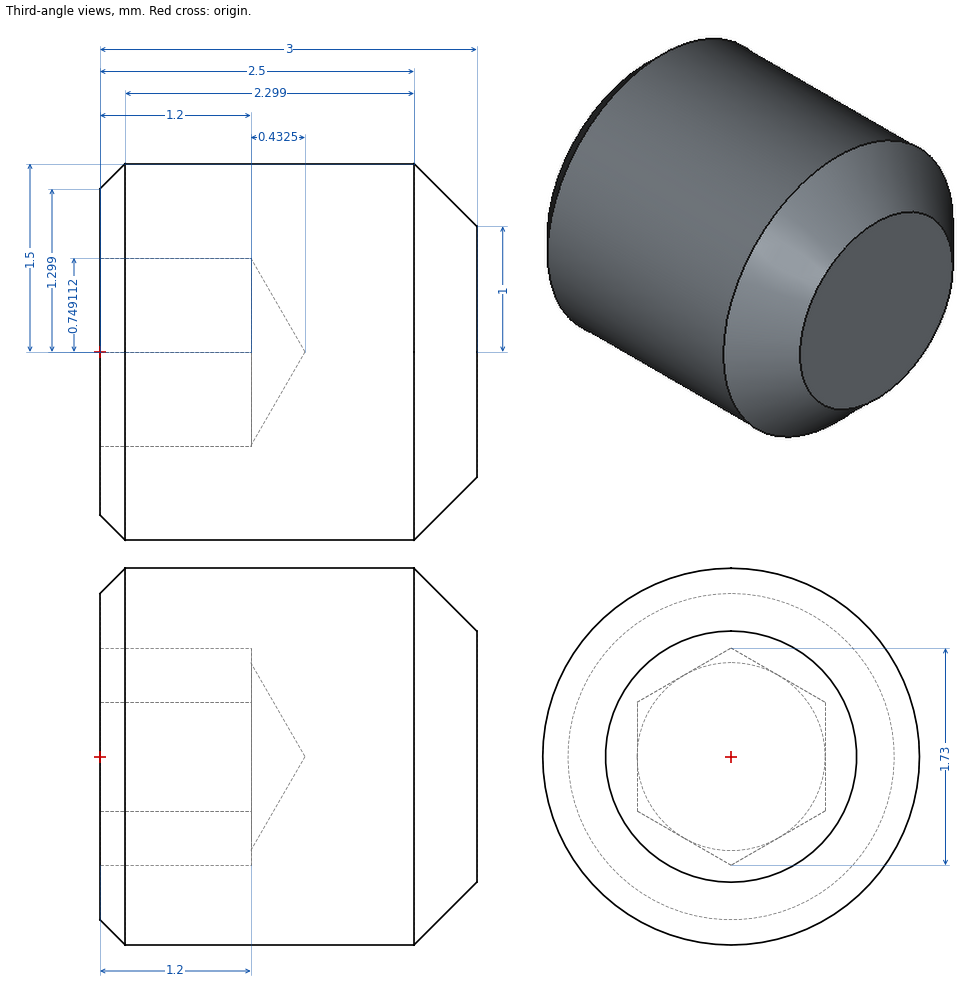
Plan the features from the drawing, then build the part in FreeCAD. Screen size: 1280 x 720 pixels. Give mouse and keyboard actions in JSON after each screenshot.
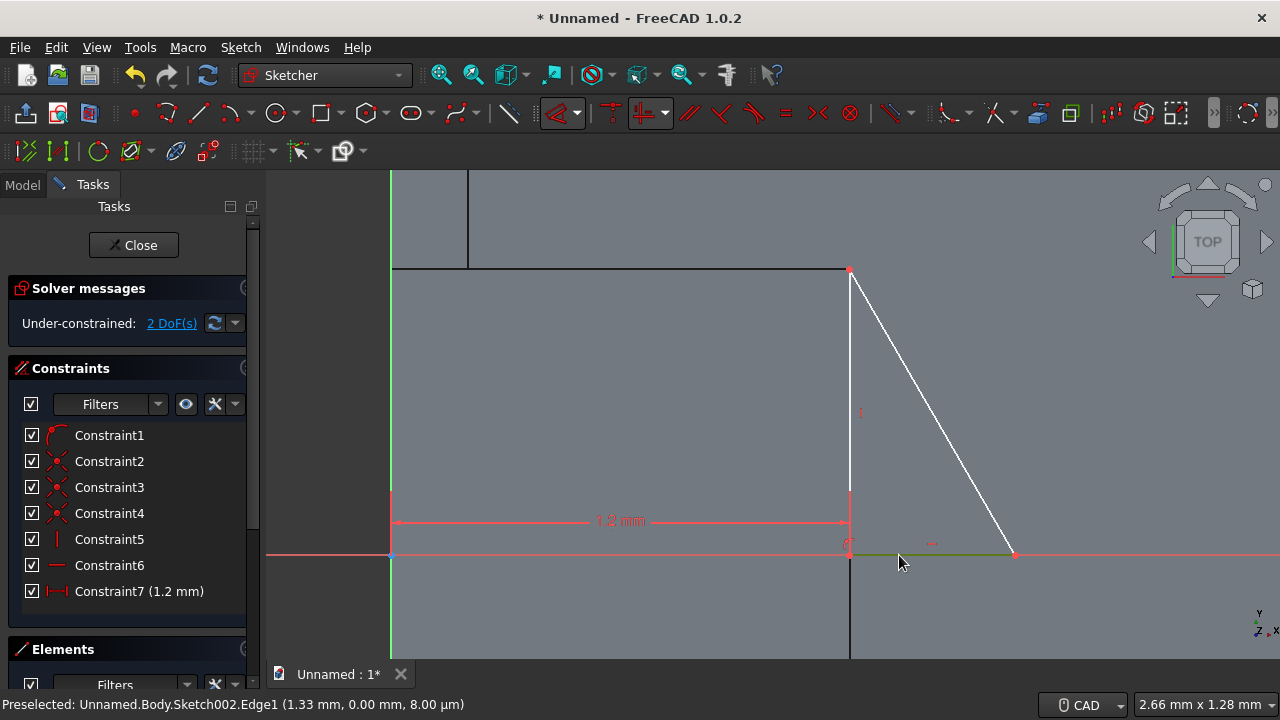
{"action": "key", "text": "l"}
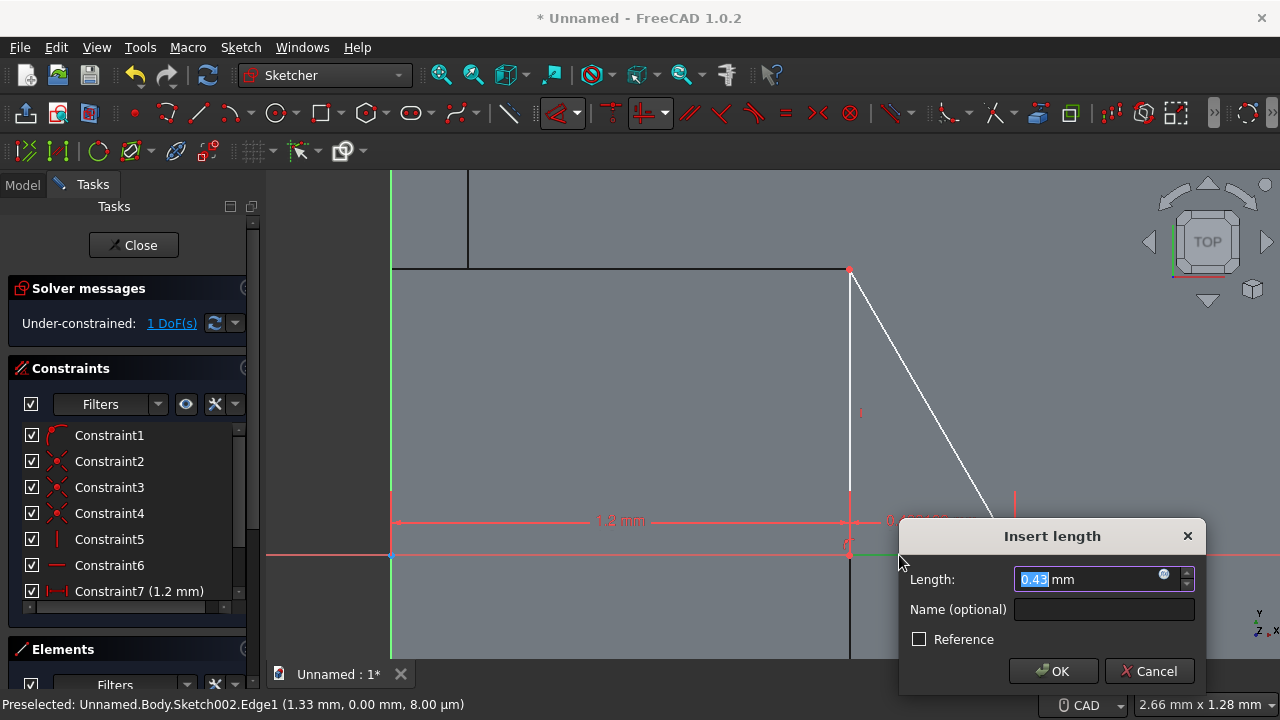
{"action": "type", "text": "0.4325"}
{"action": "key", "text": "Return"}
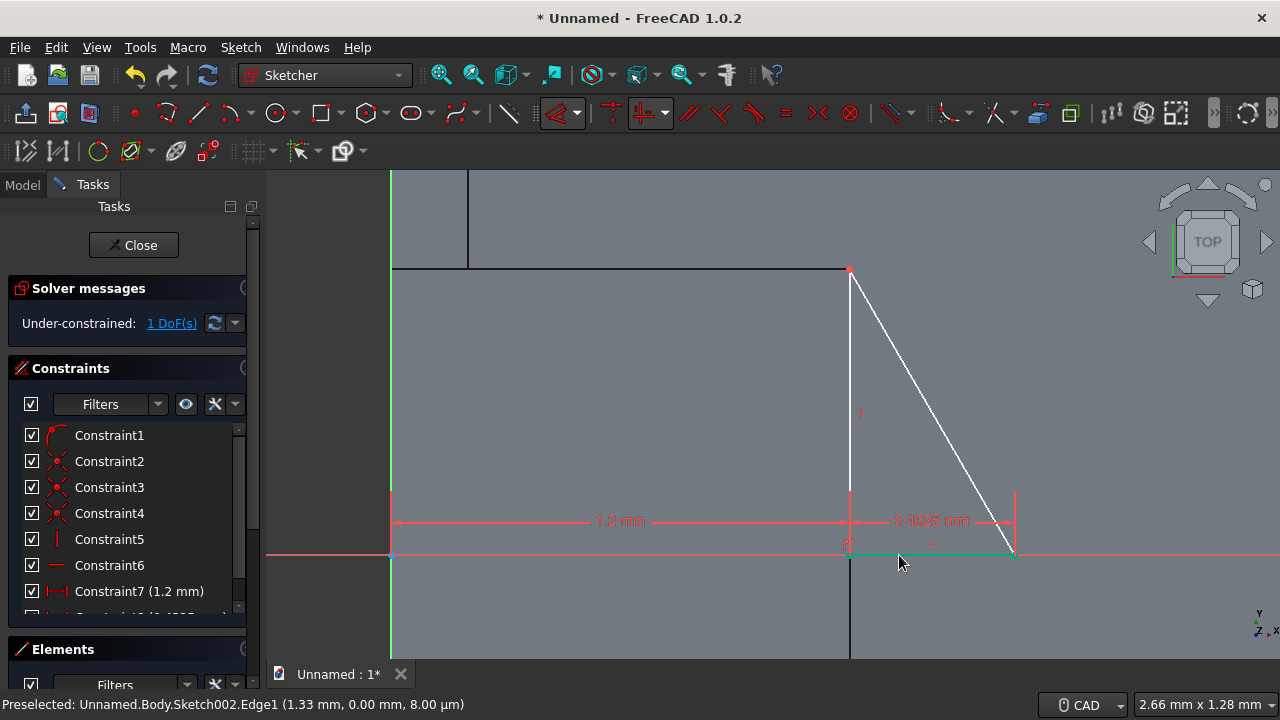
{"action": "left_click", "coordinate": [850, 356]}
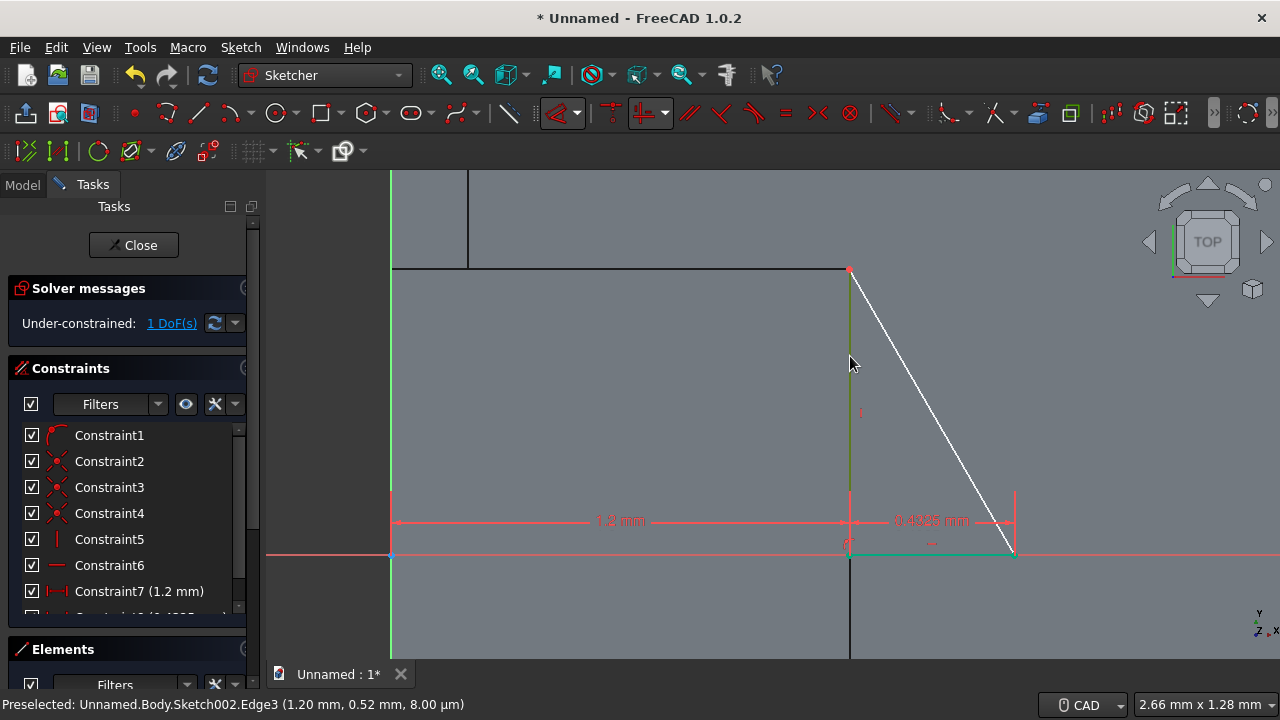
{"action": "key", "text": "i"}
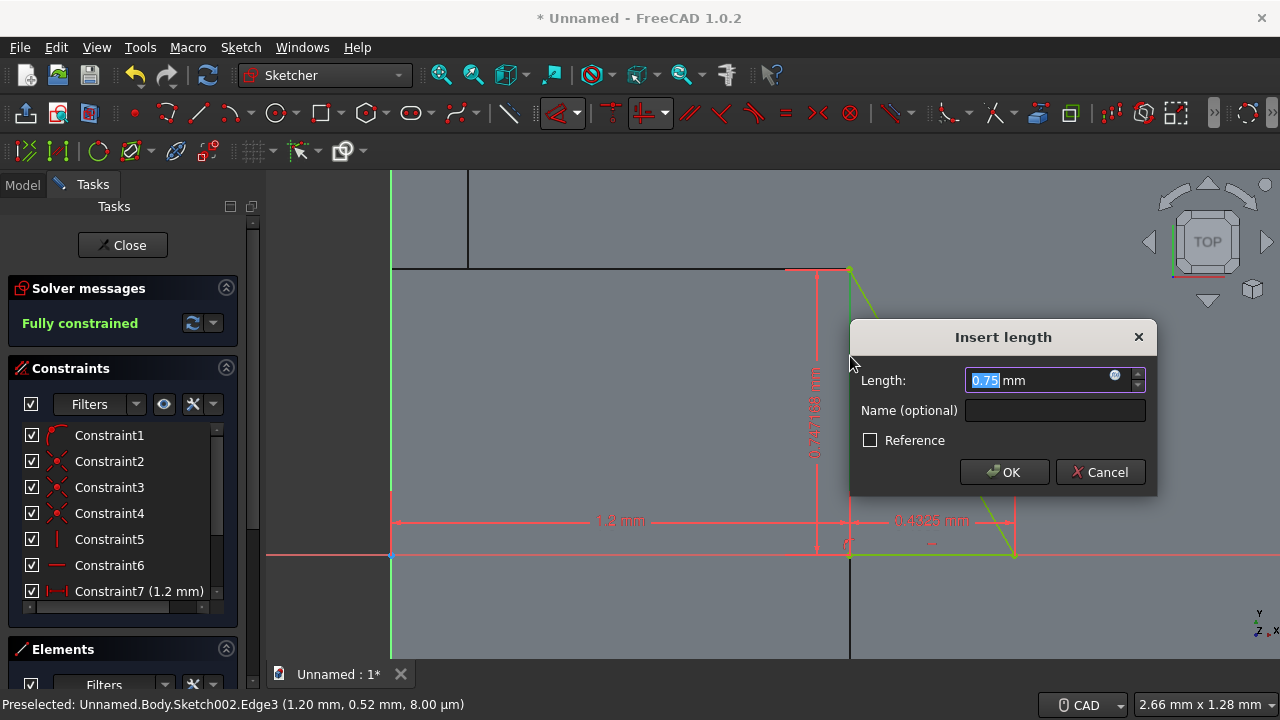
{"action": "type", "text": "0.749112"}
{"action": "key", "text": "Return"}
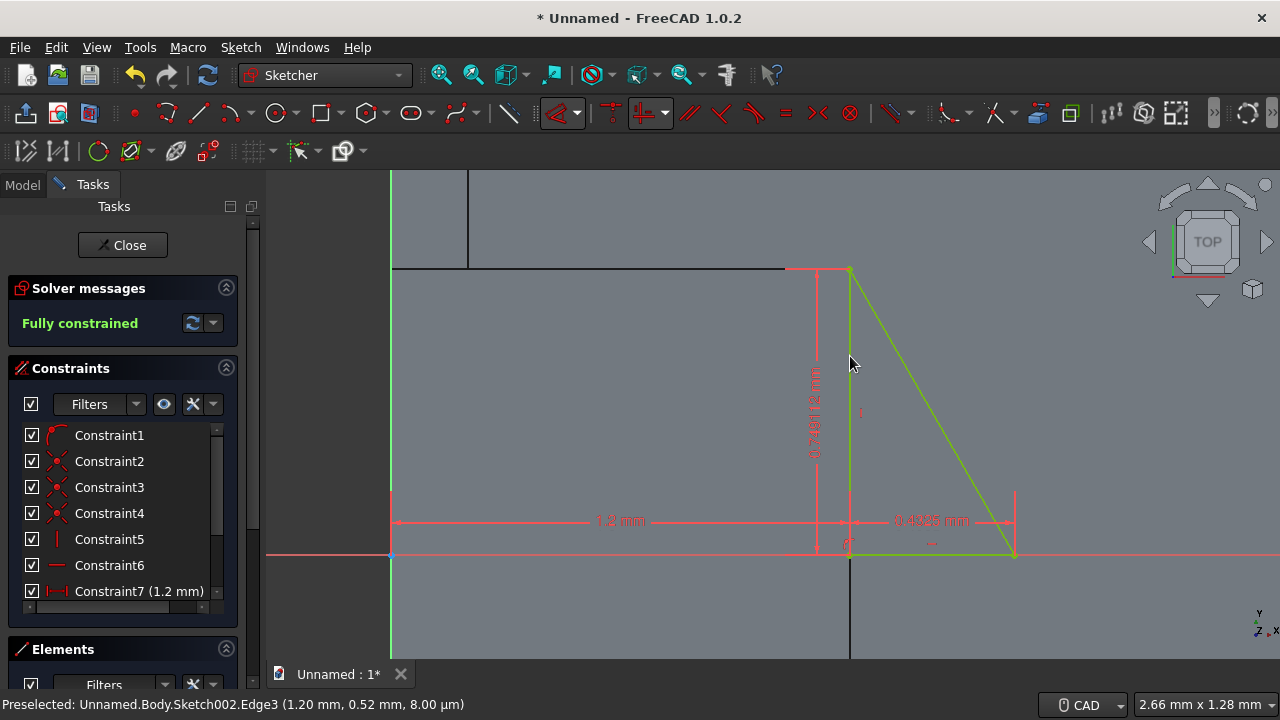
{"action": "left_click", "coordinate": [123, 245]}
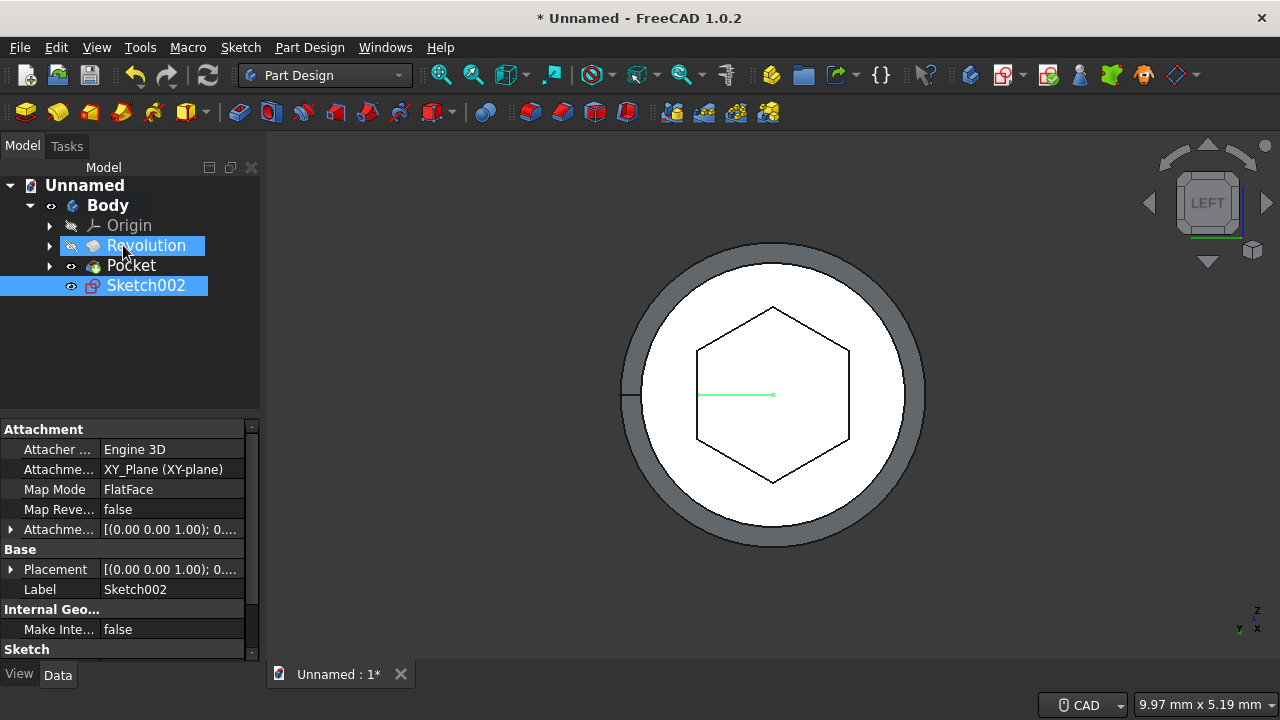
{"action": "left_click", "coordinate": [304, 112]}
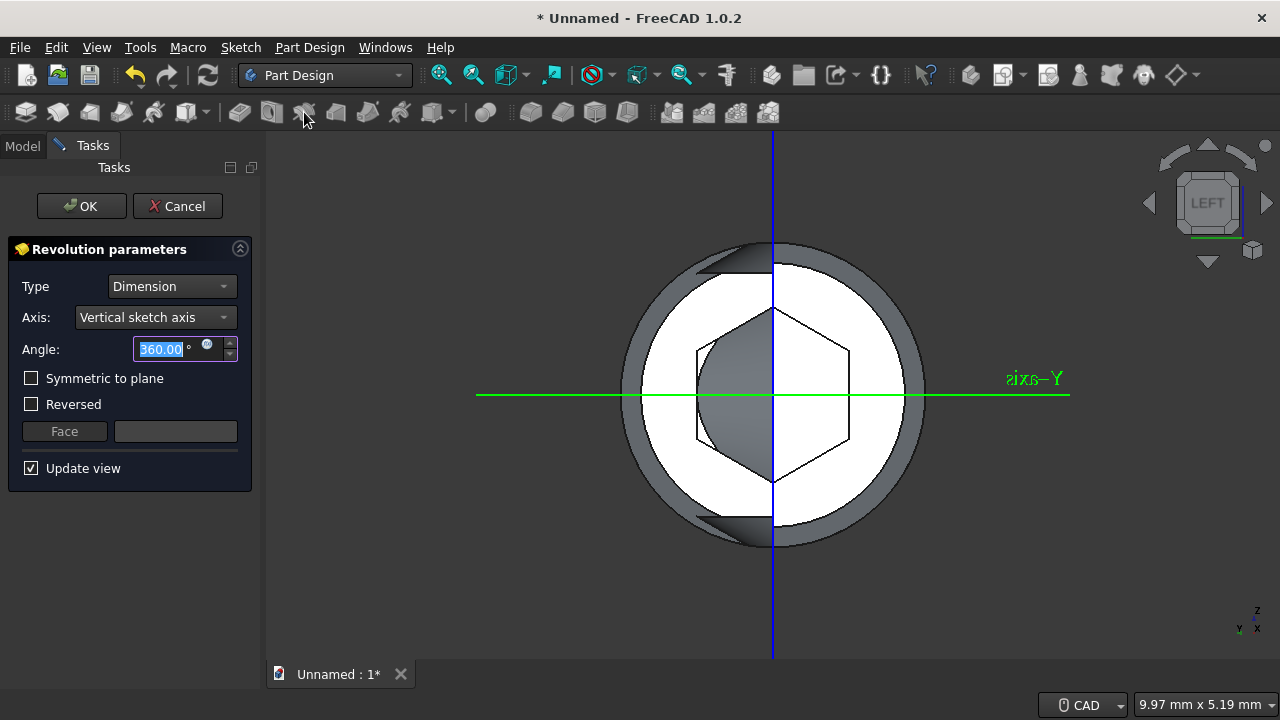
{"action": "left_click", "coordinate": [156, 318]}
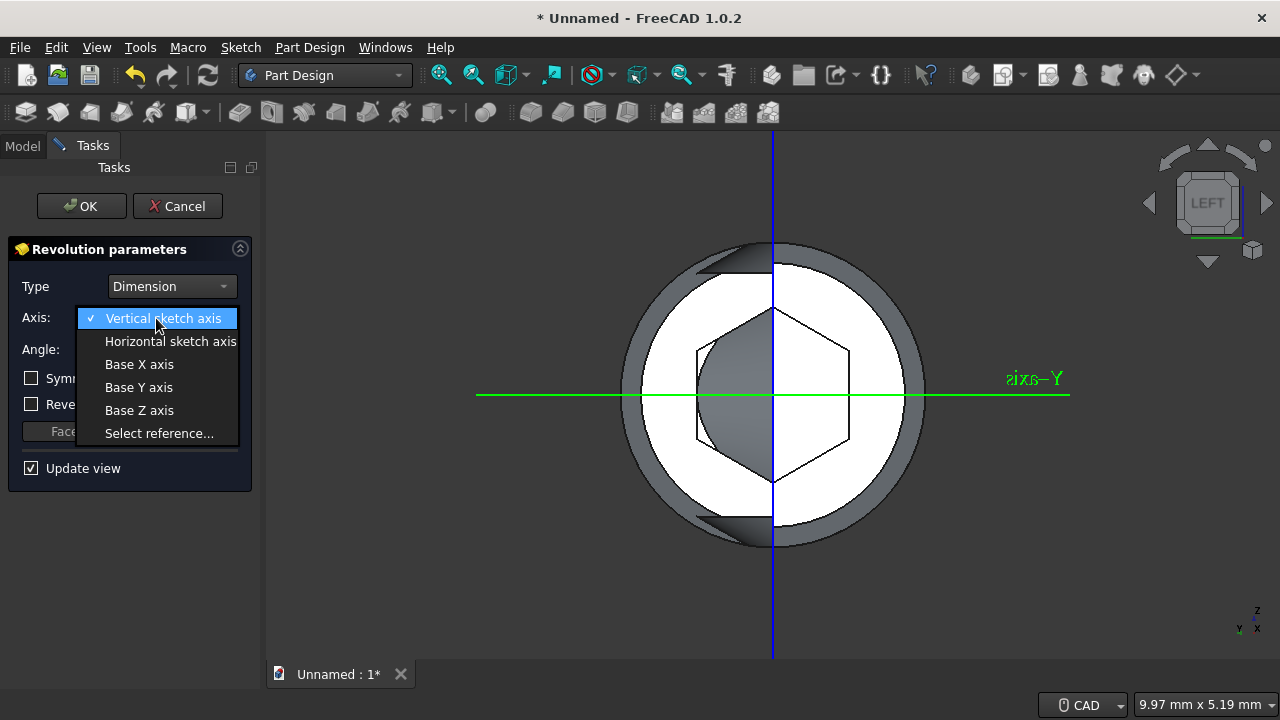
{"action": "left_click", "coordinate": [156, 342]}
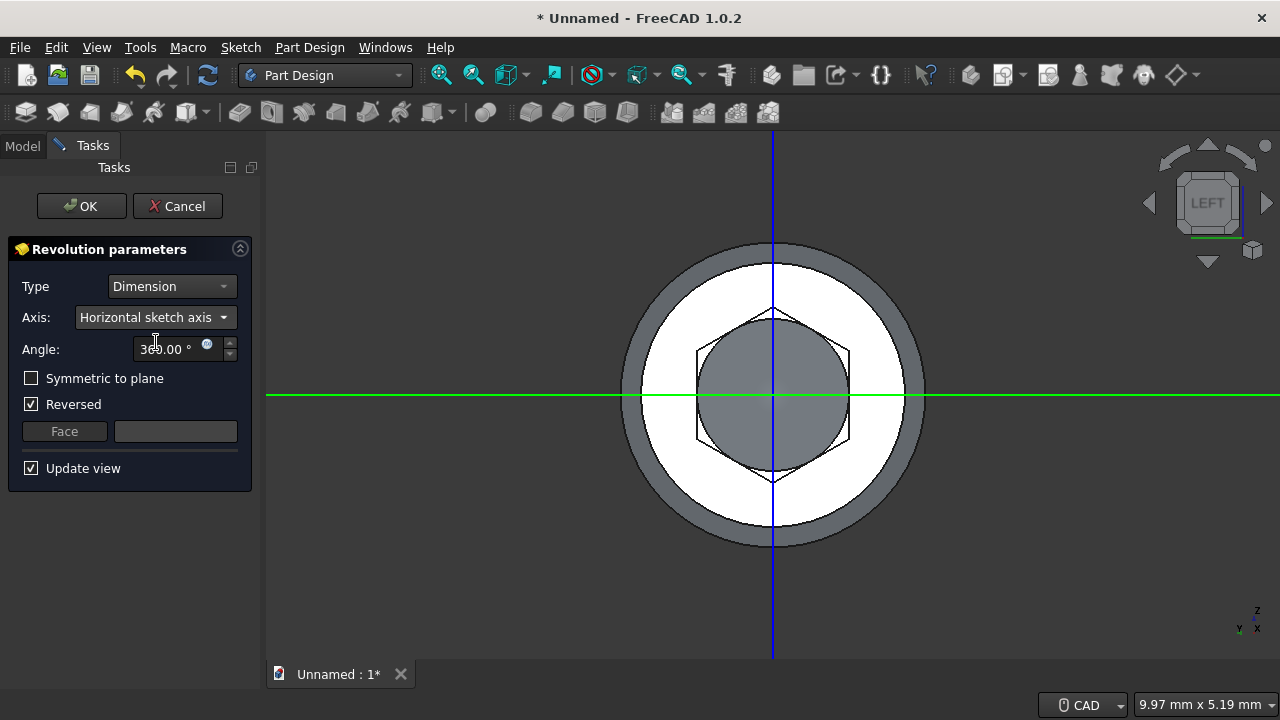
{"action": "left_click", "coordinate": [82, 206]}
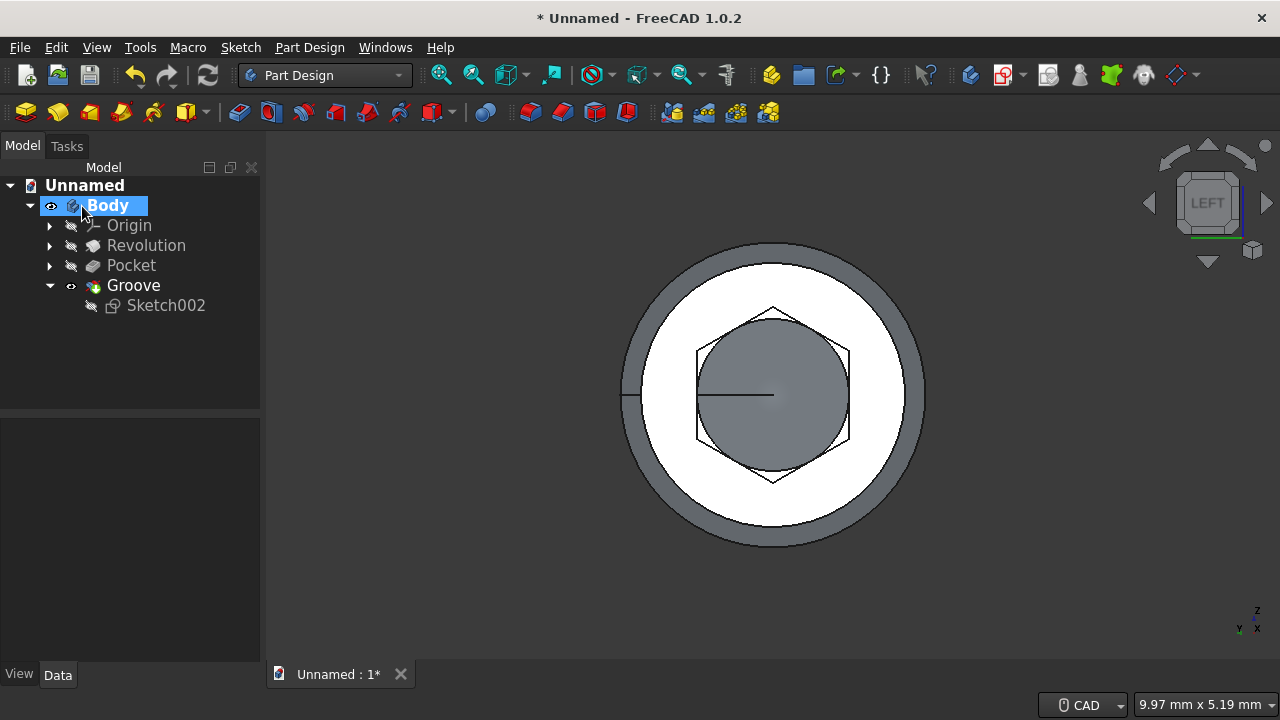
{"action": "key", "text": "0"}